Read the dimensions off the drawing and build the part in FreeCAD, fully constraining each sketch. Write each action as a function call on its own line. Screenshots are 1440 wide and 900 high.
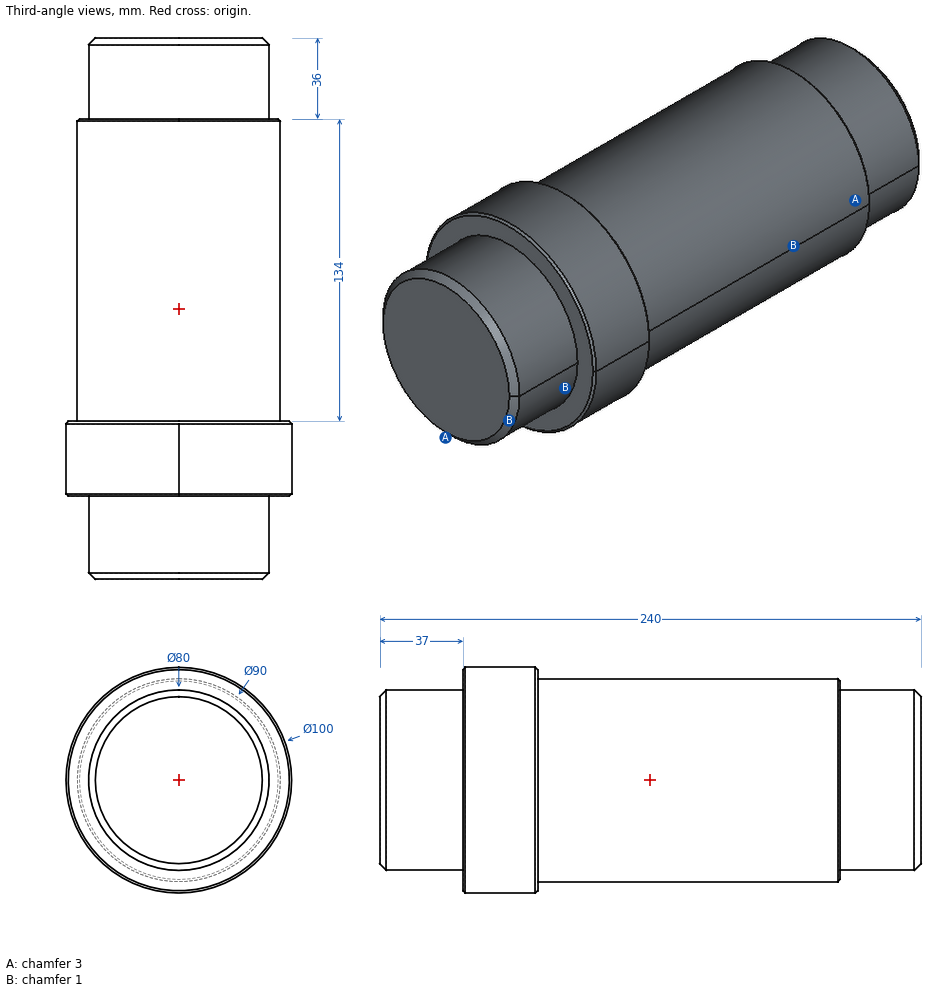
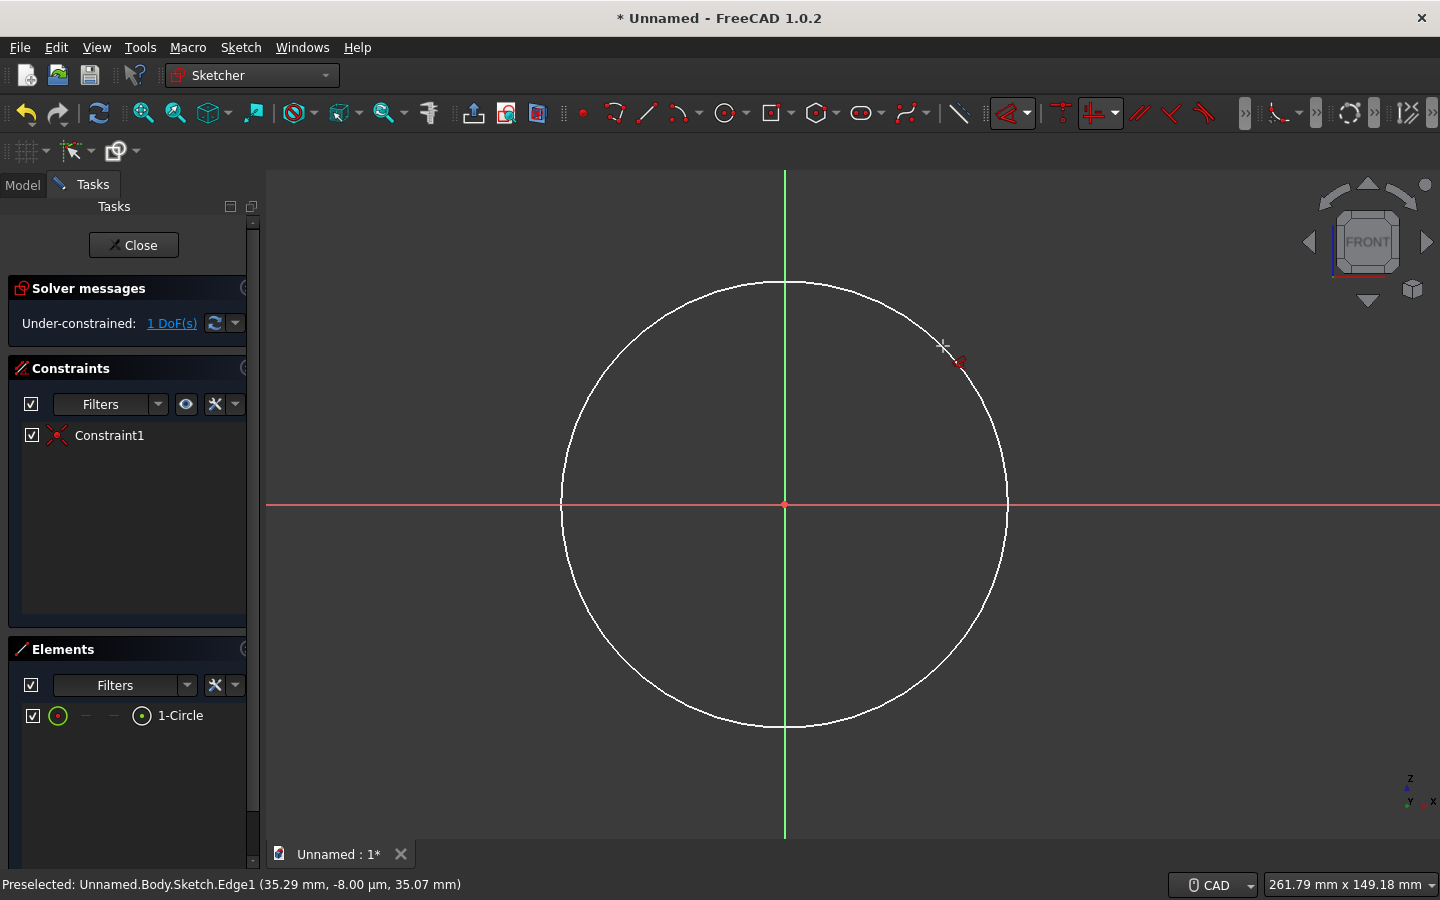
click(942, 346)
click(965, 323)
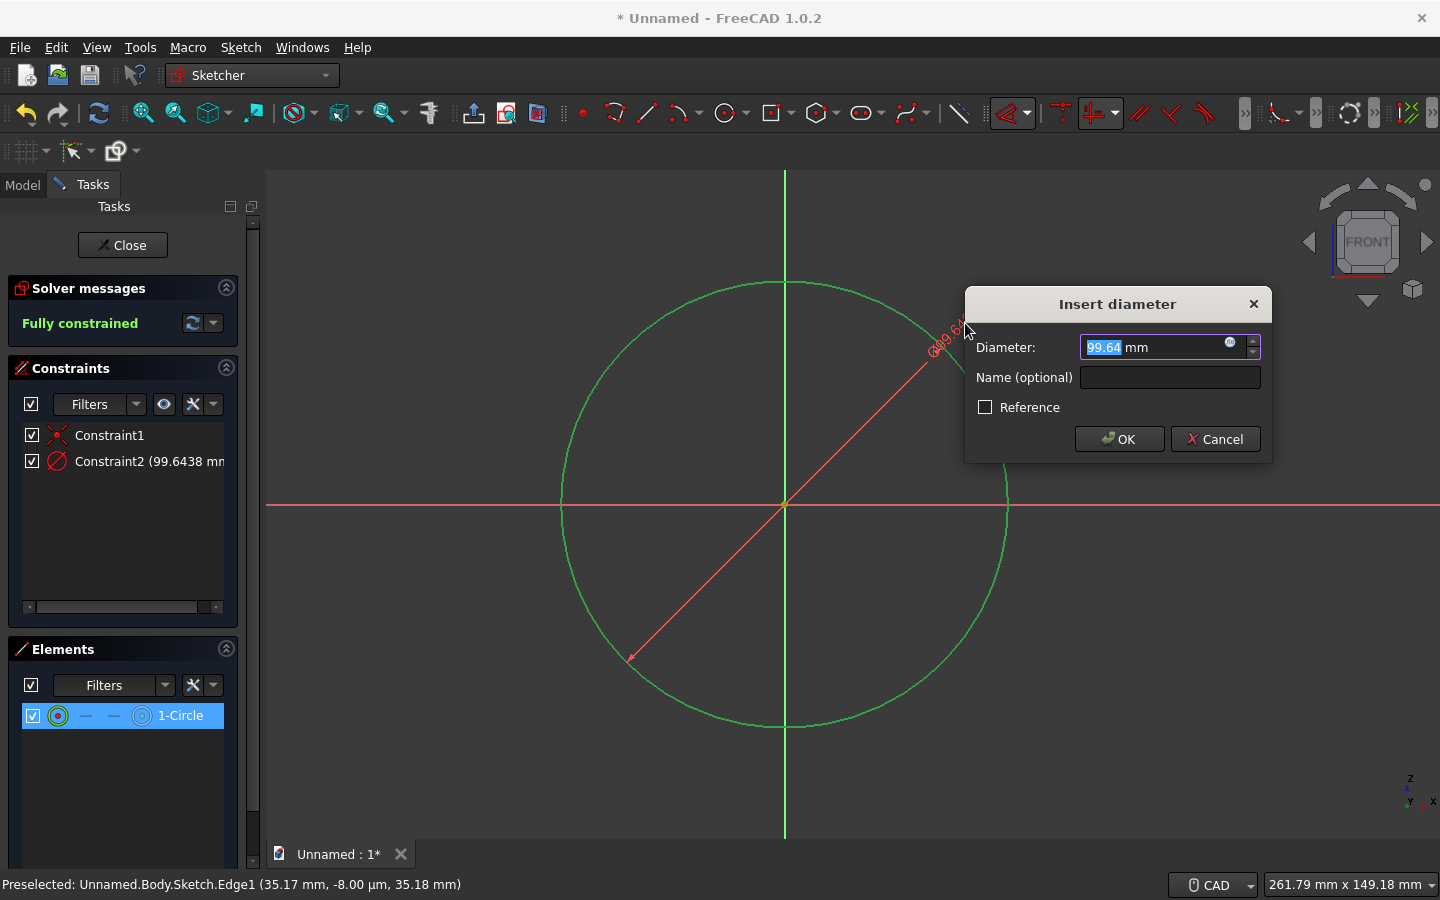
text(100)
key(Return)
key(Escape)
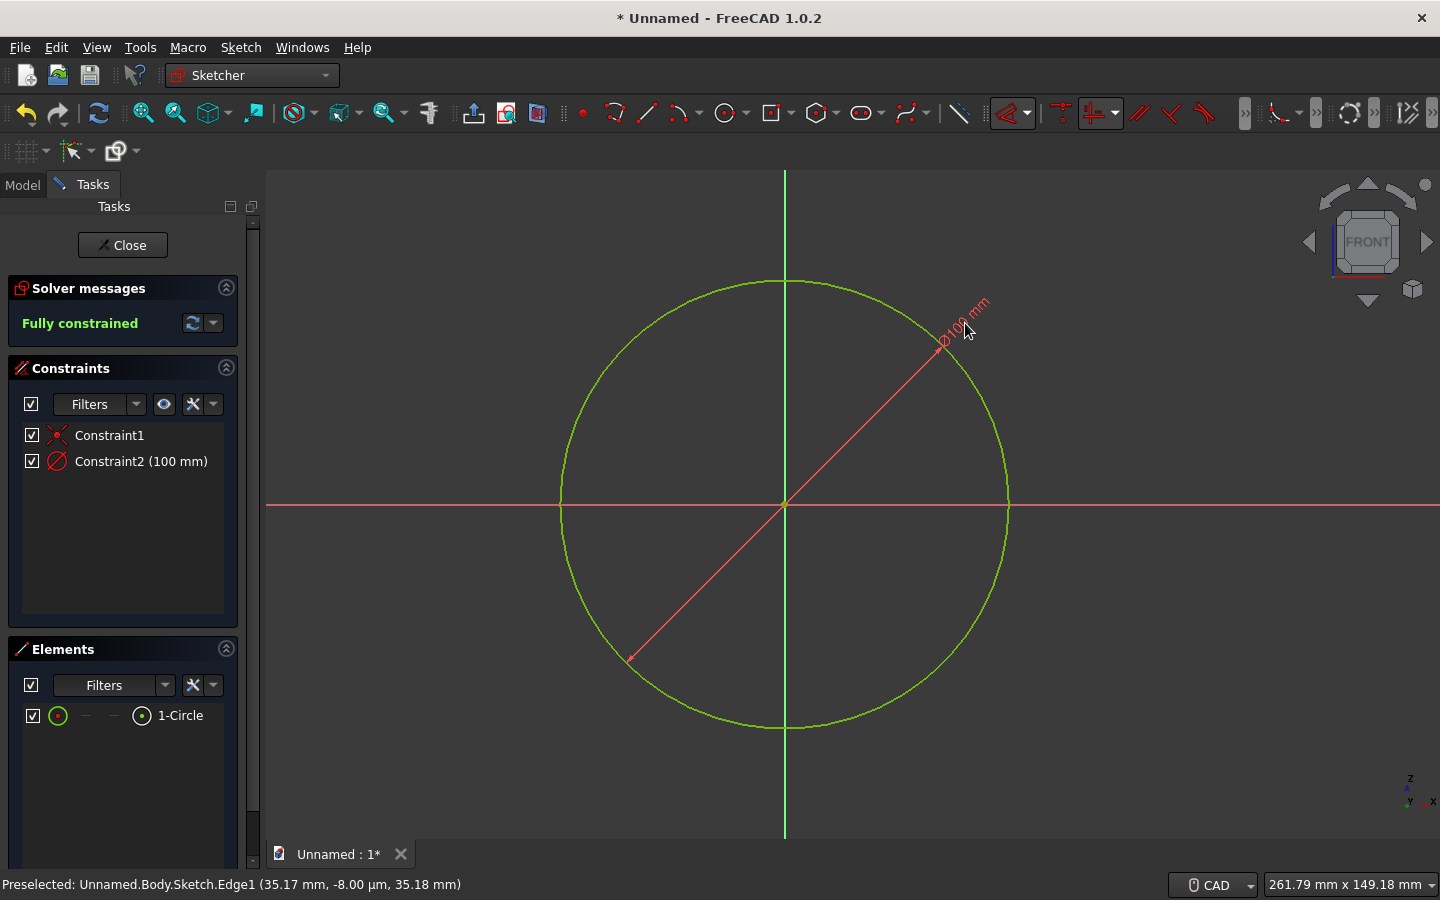
click(123, 245)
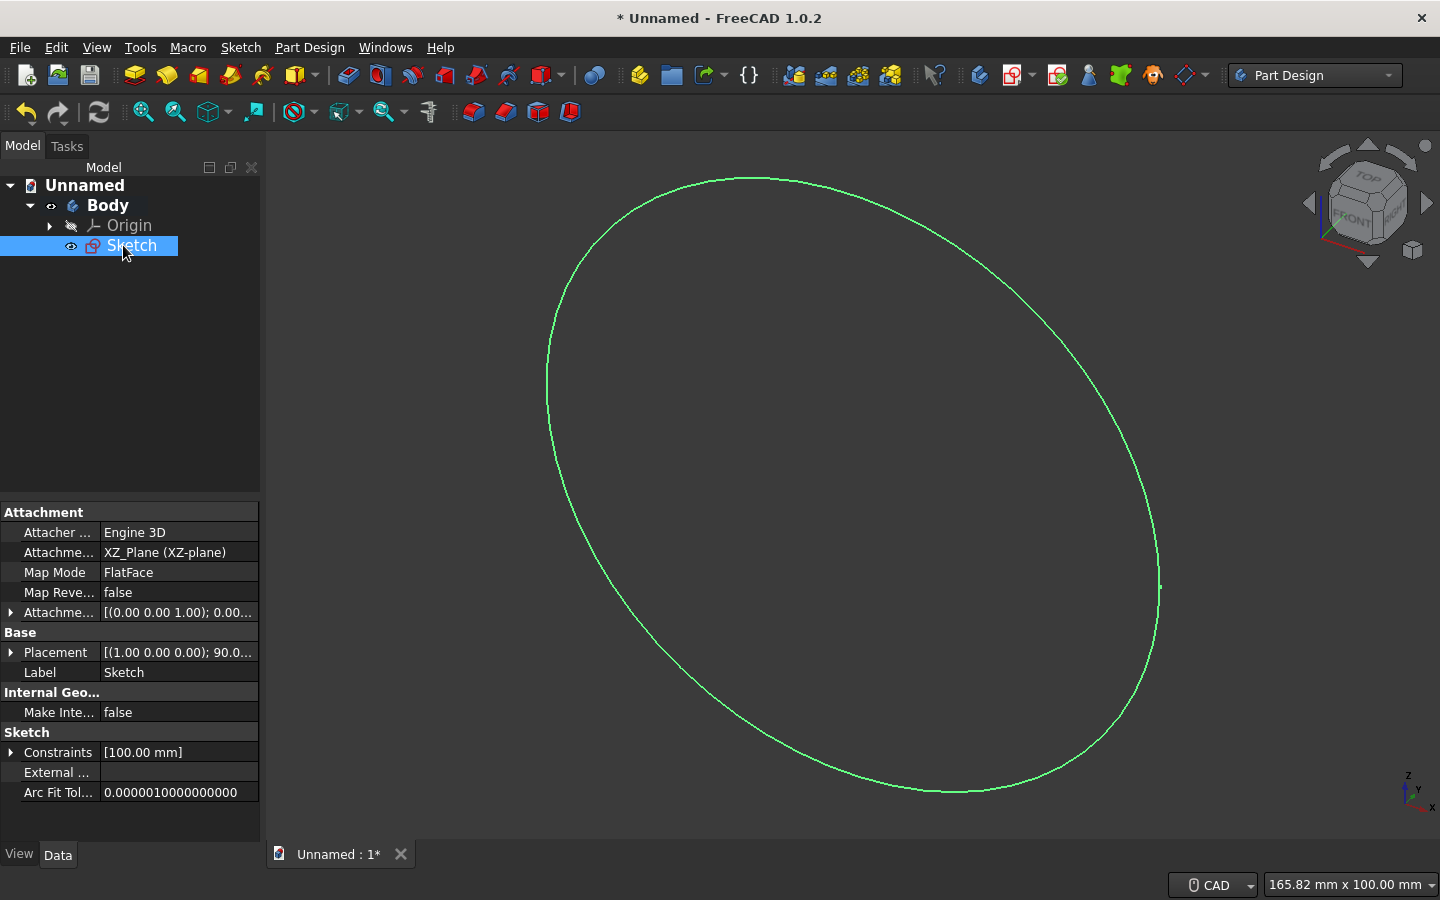
click(136, 76)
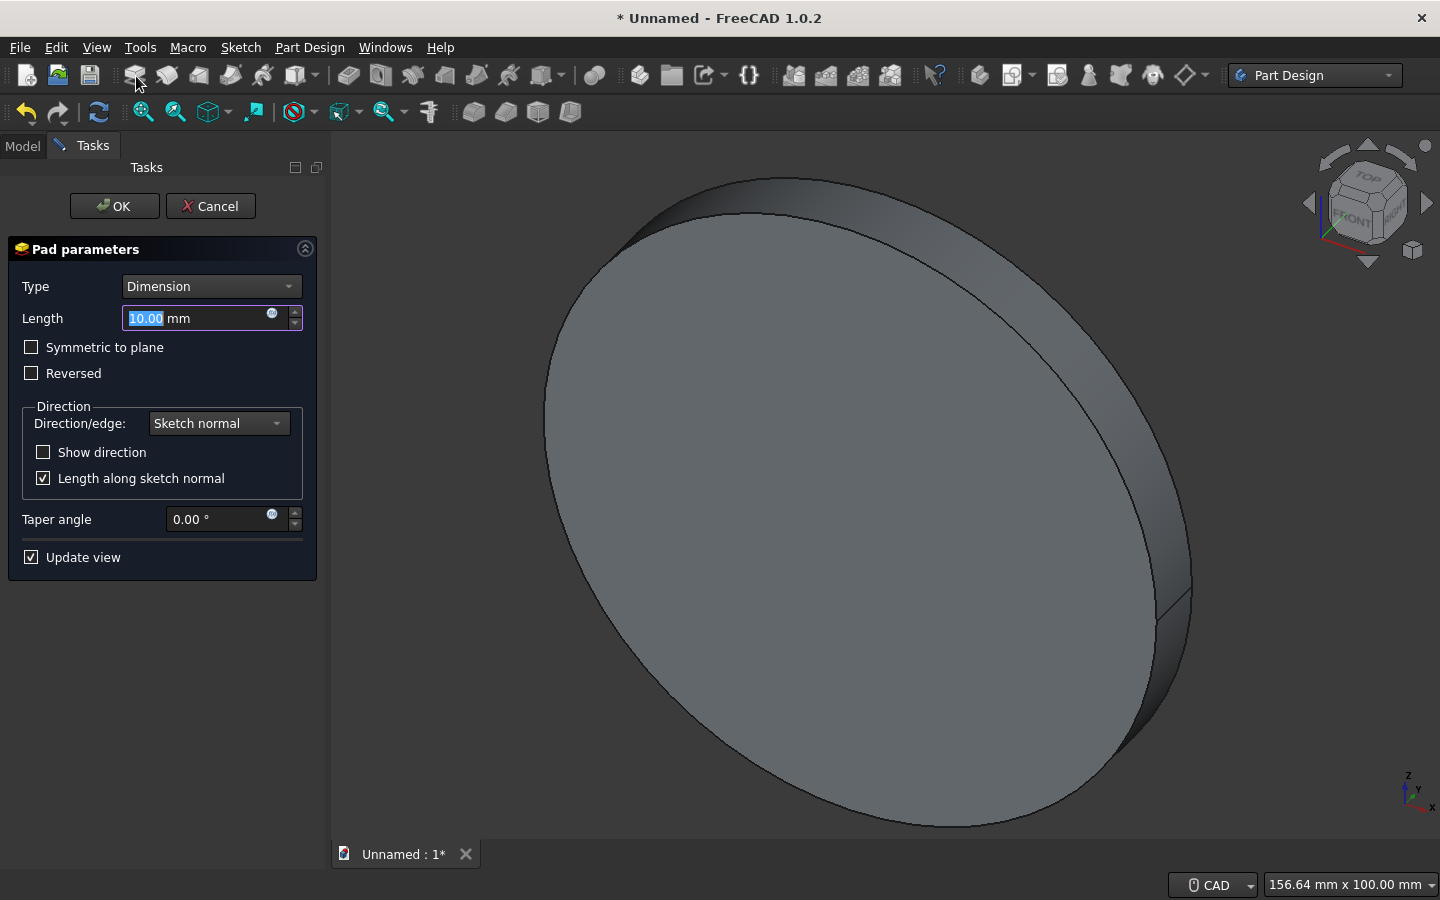
text(240)
key(Tab)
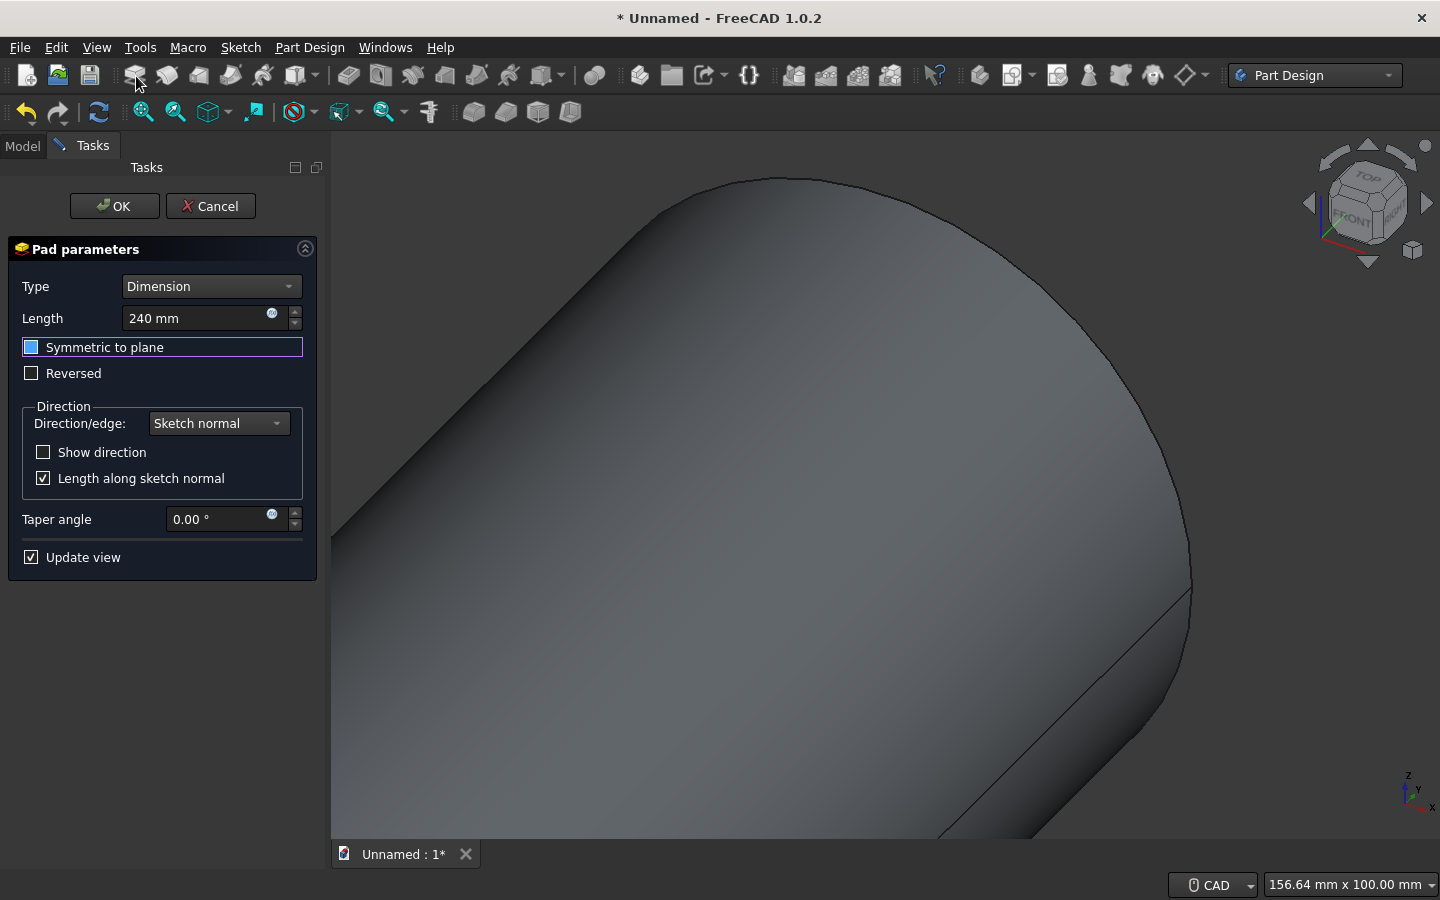
click(30, 347)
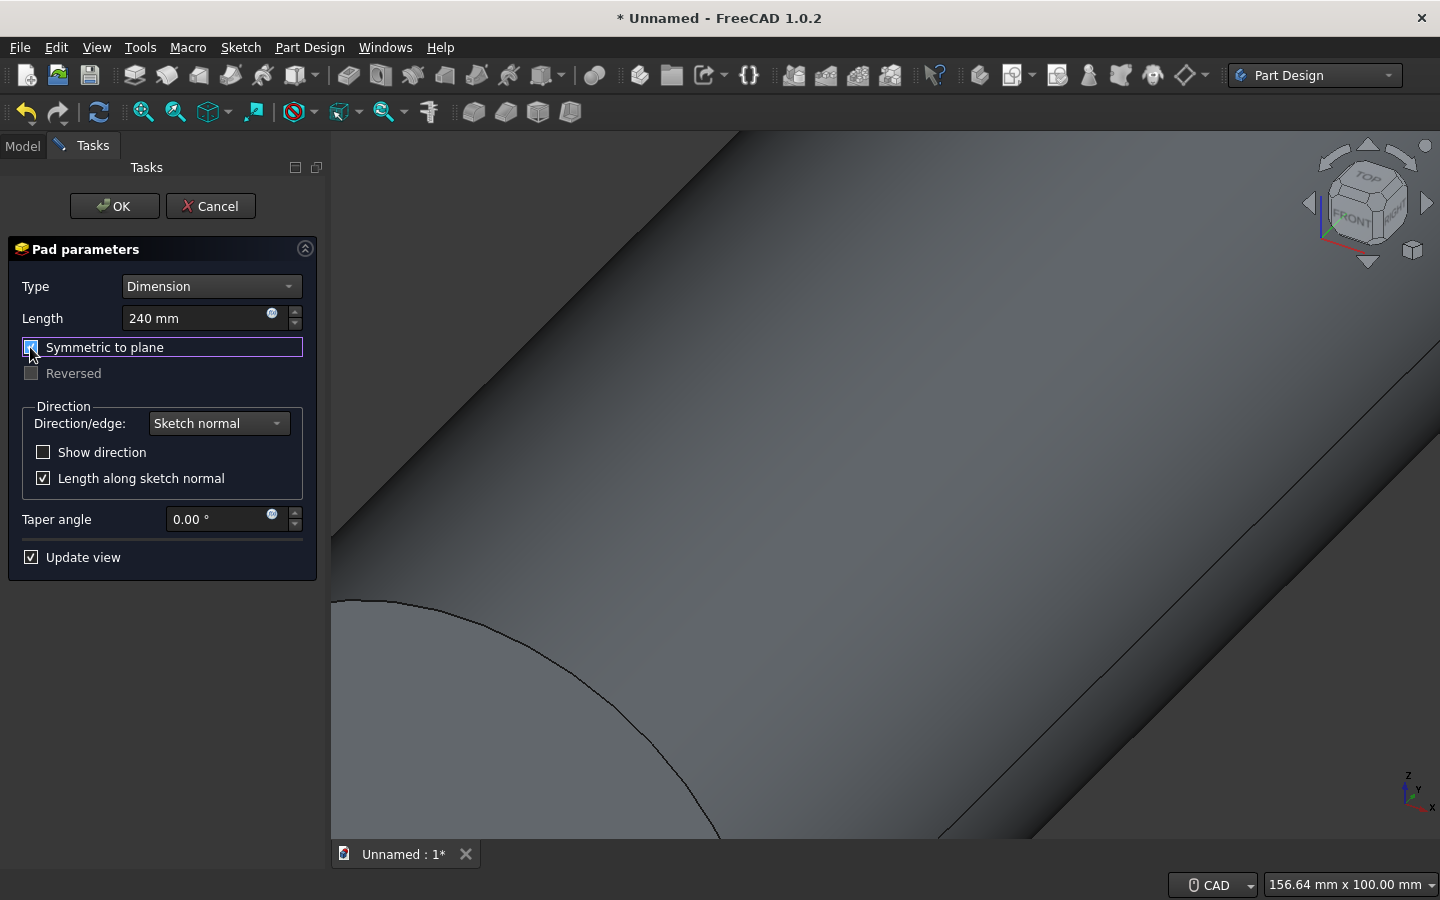
click(115, 206)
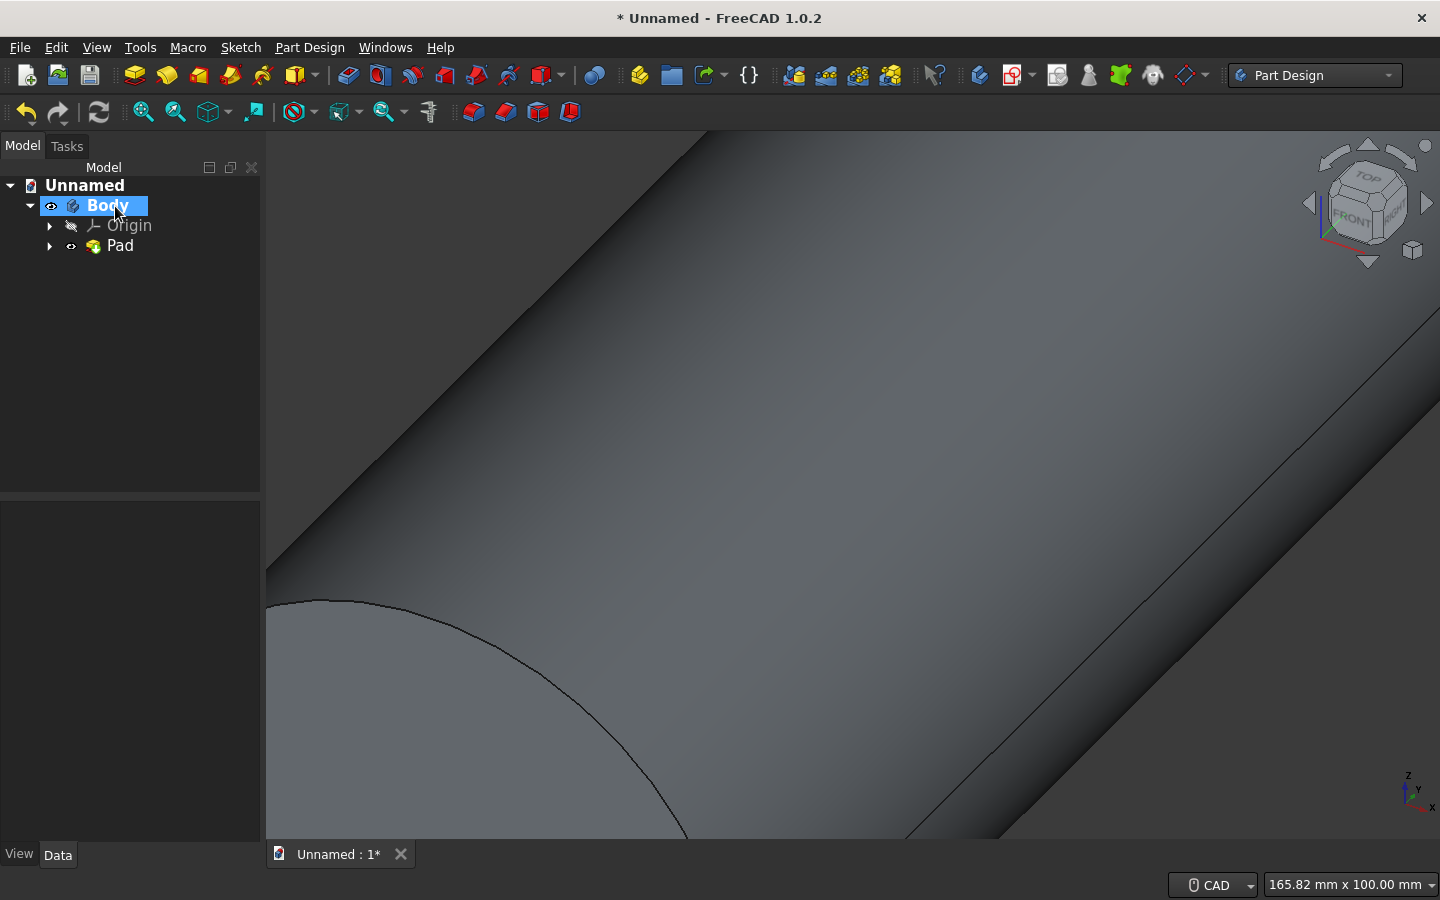
click(144, 112)